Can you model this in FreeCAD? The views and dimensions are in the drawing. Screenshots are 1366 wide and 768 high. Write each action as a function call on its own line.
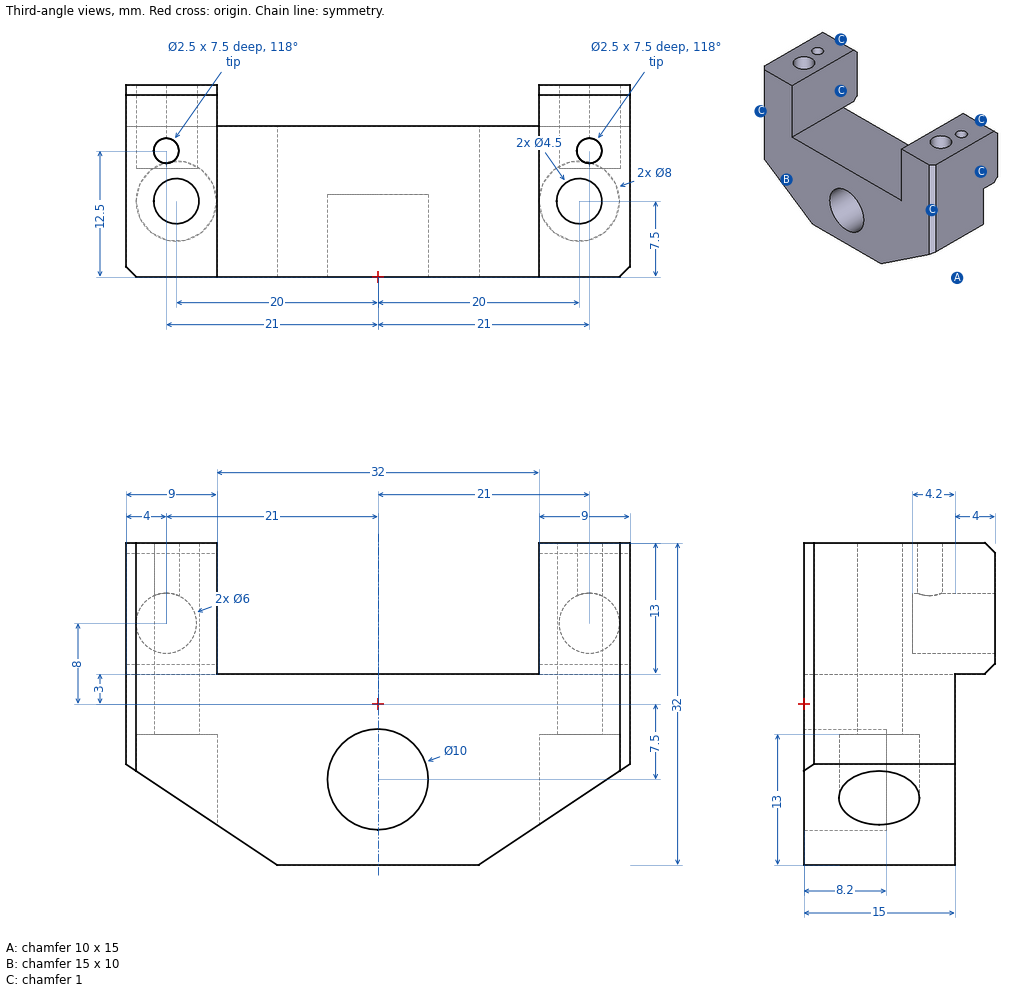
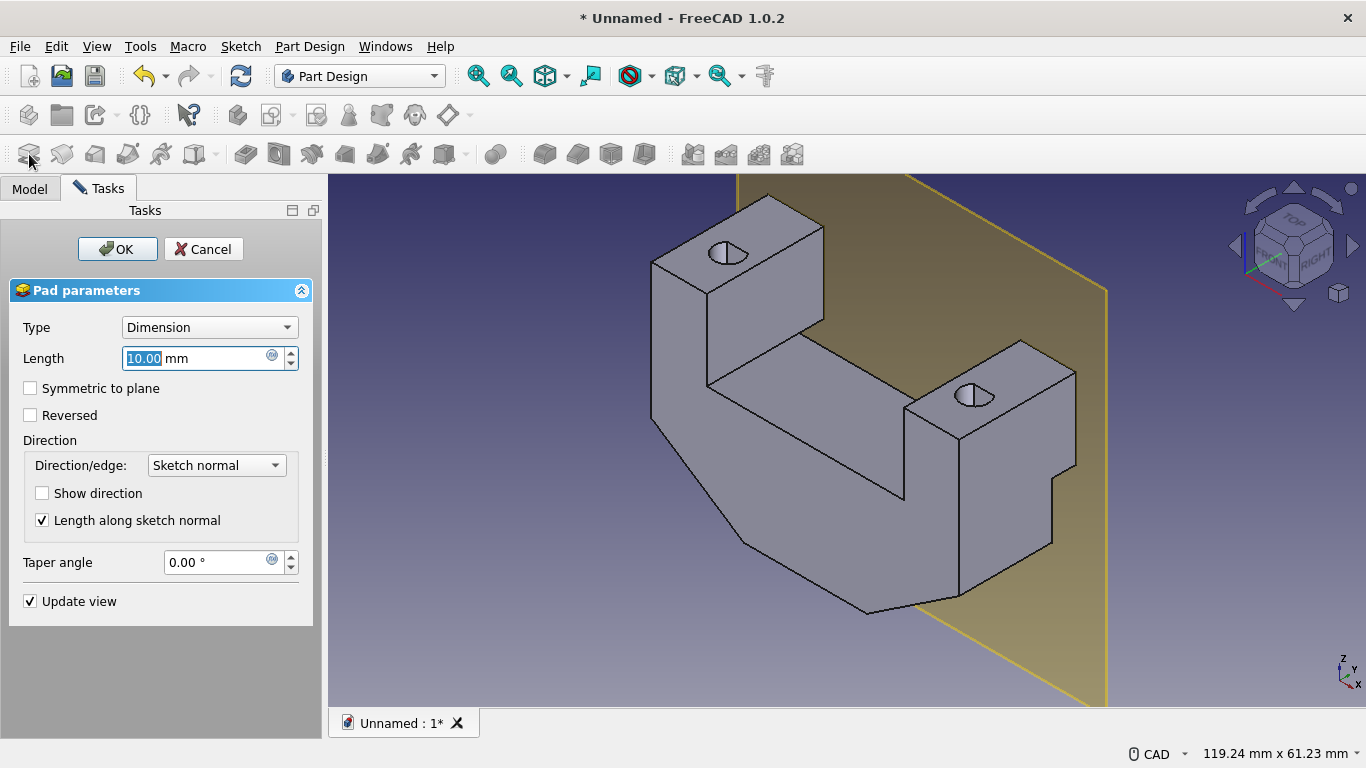
text(4)
key(Tab)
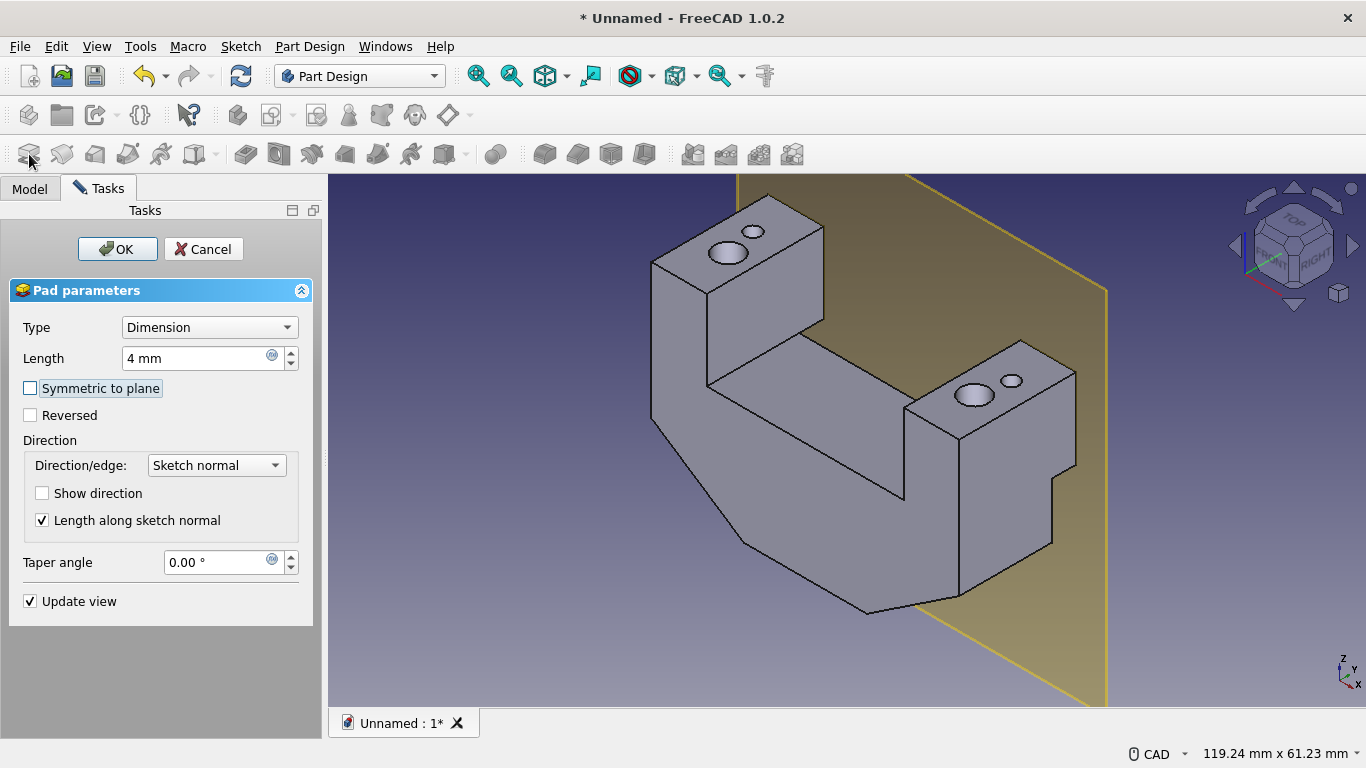
click(118, 249)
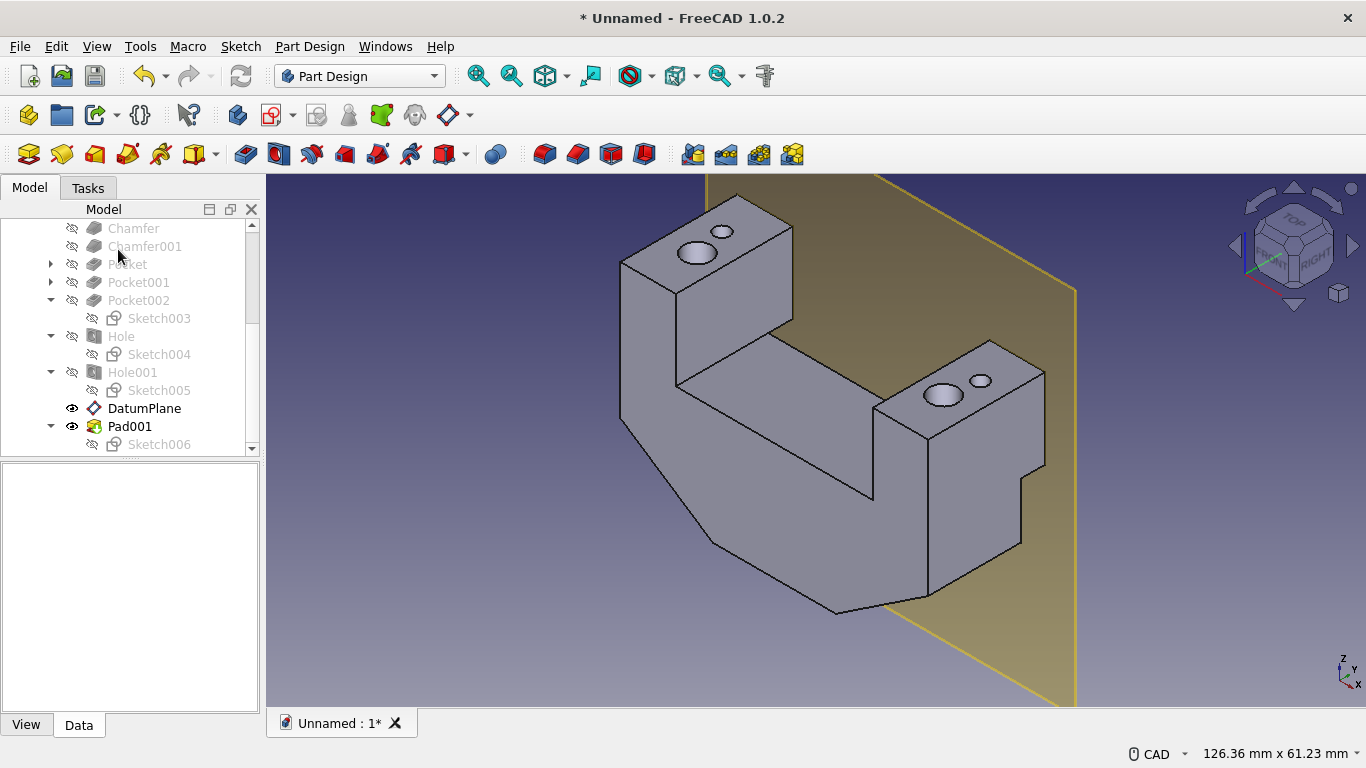
click(117, 408)
key(space)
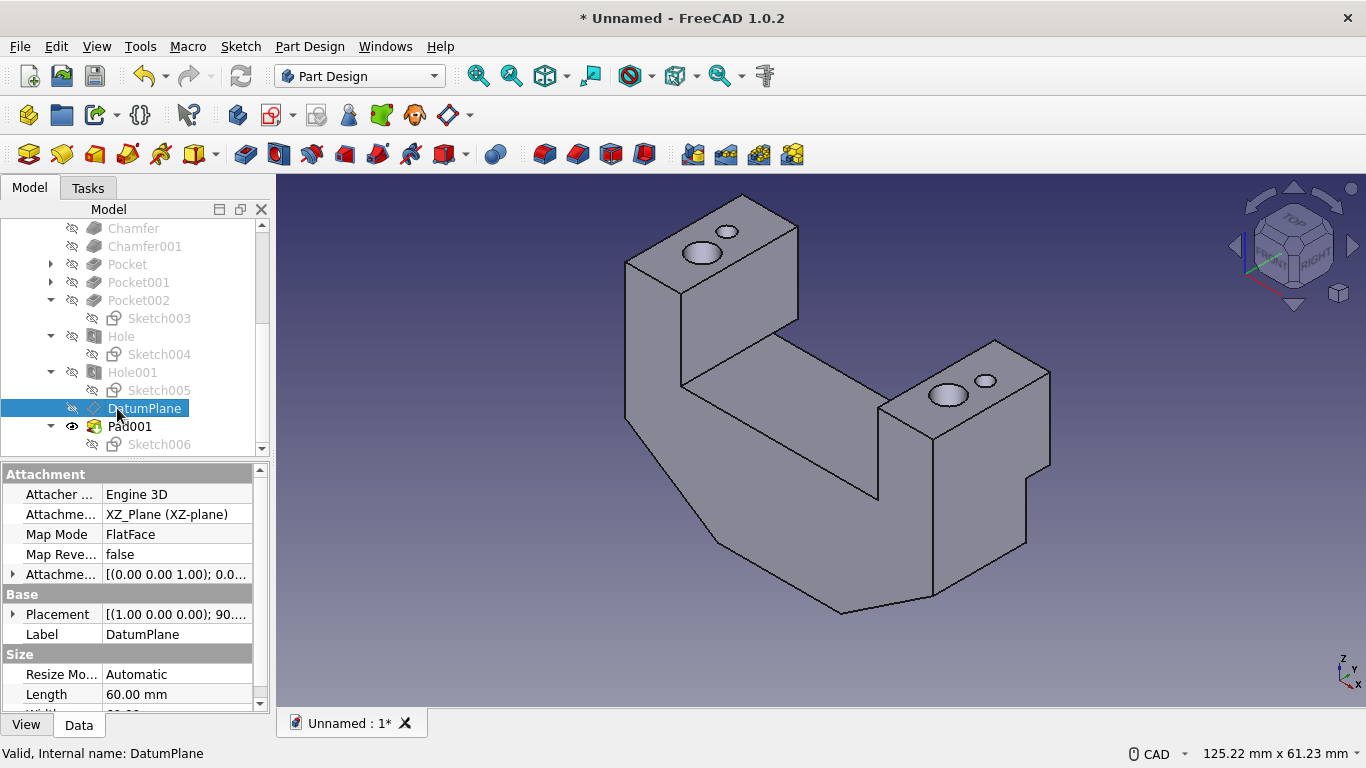
click(823, 521)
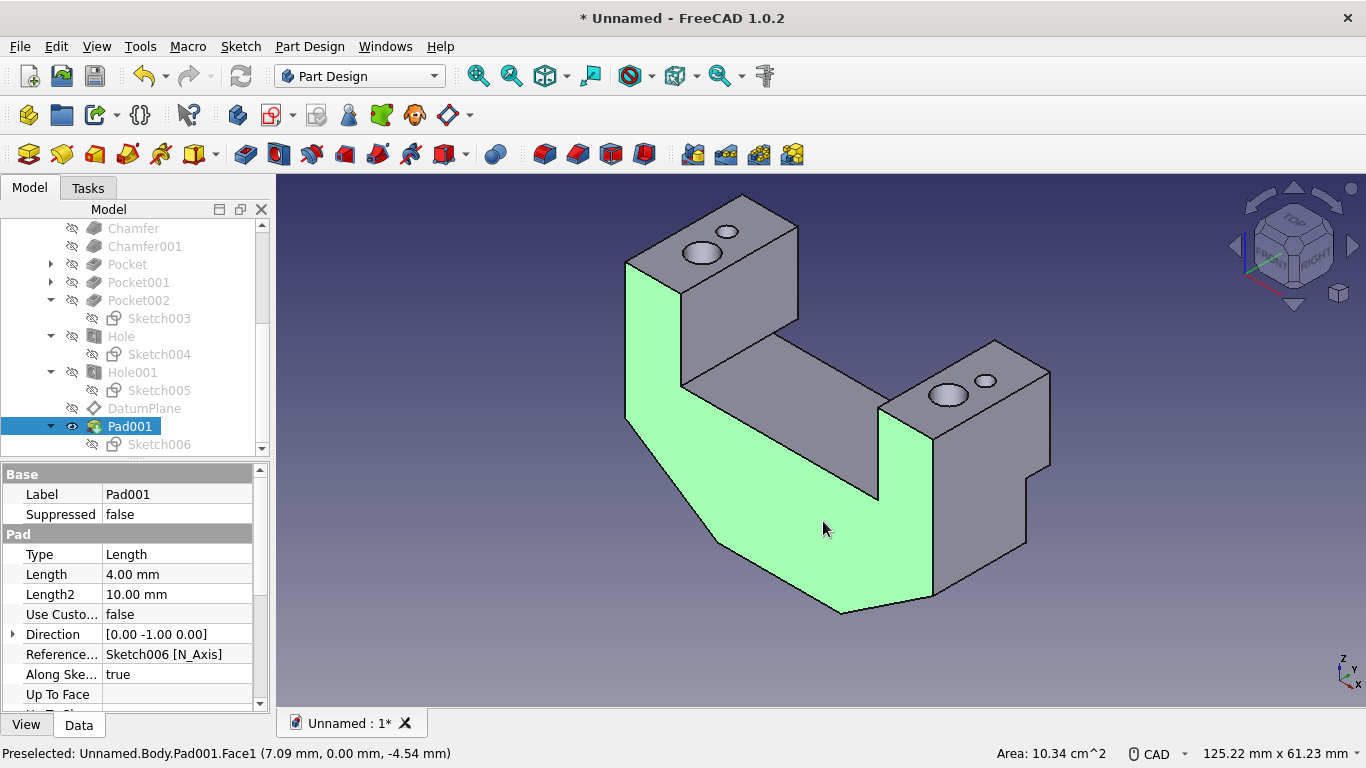
click(270, 116)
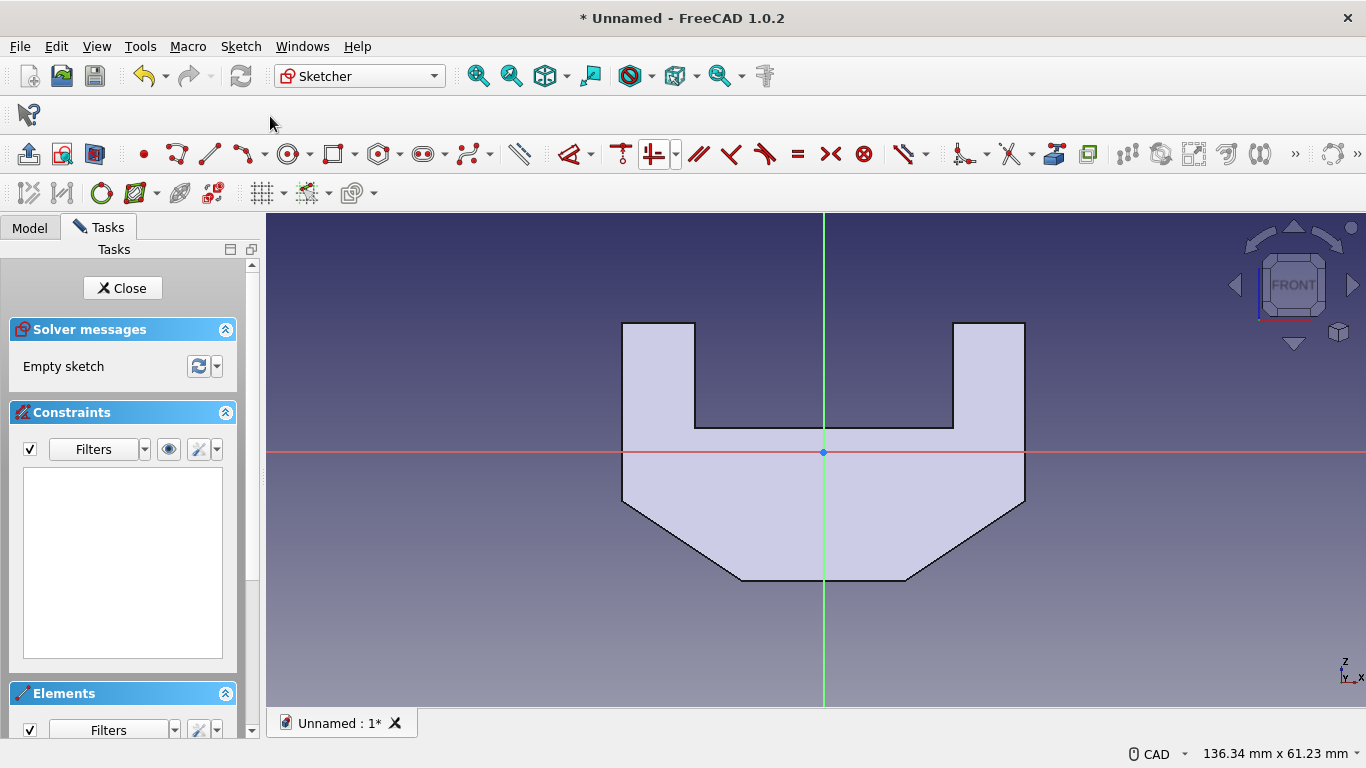
scroll(856, 521, up, 6)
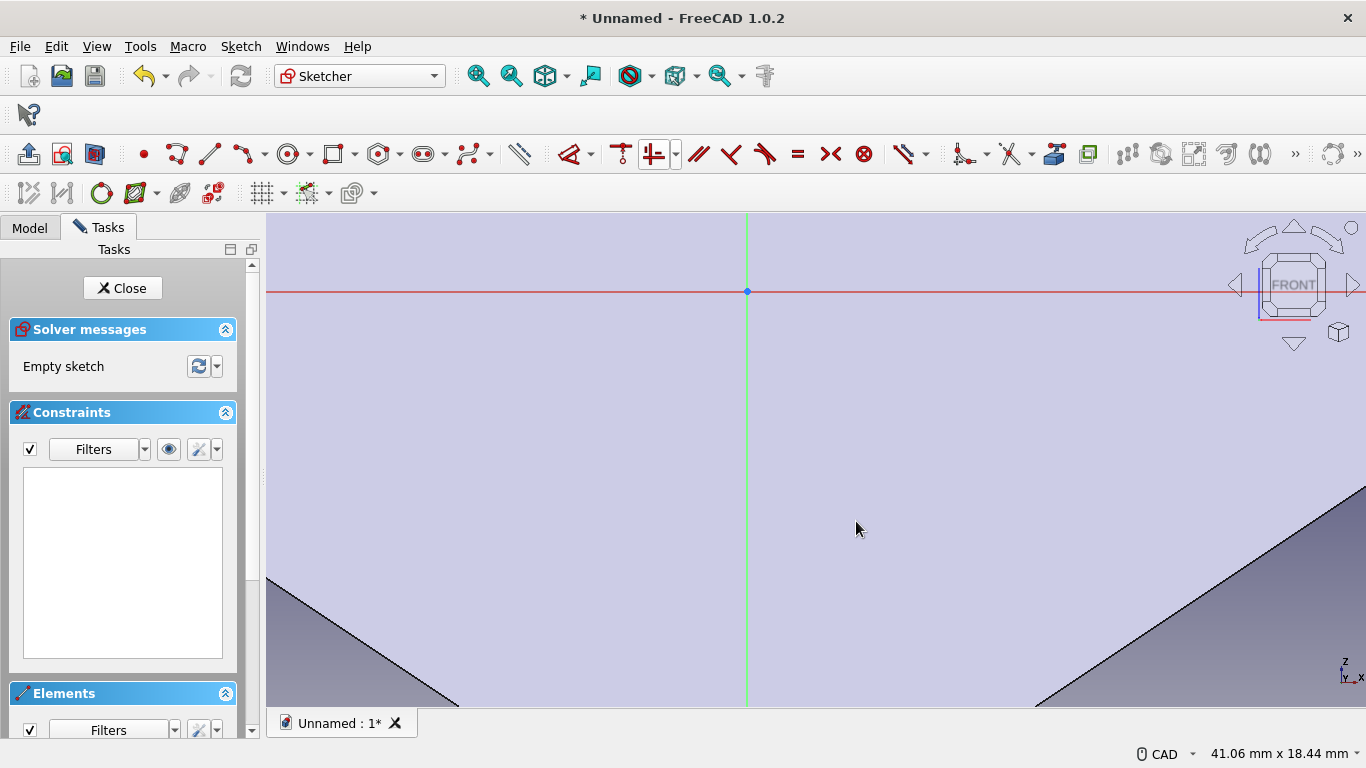
click(288, 154)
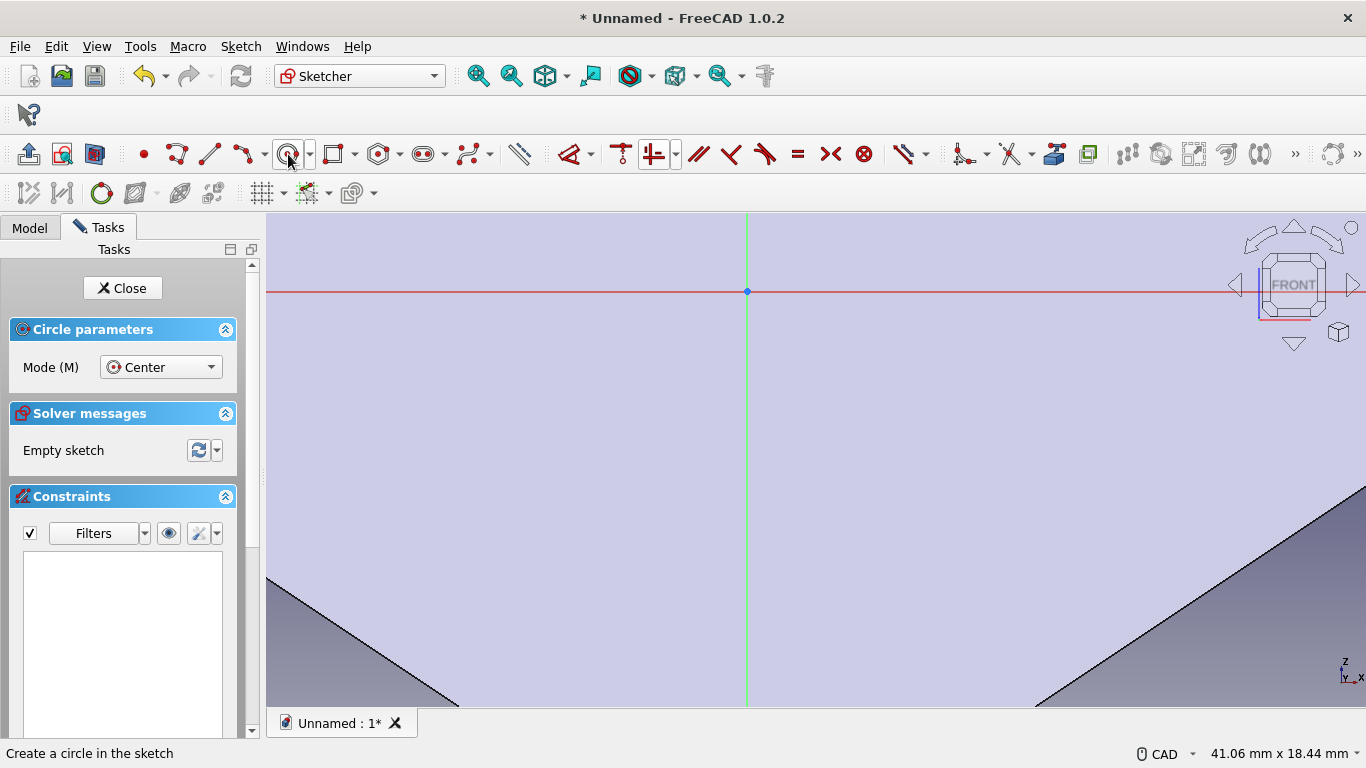
click(747, 493)
move(842, 398)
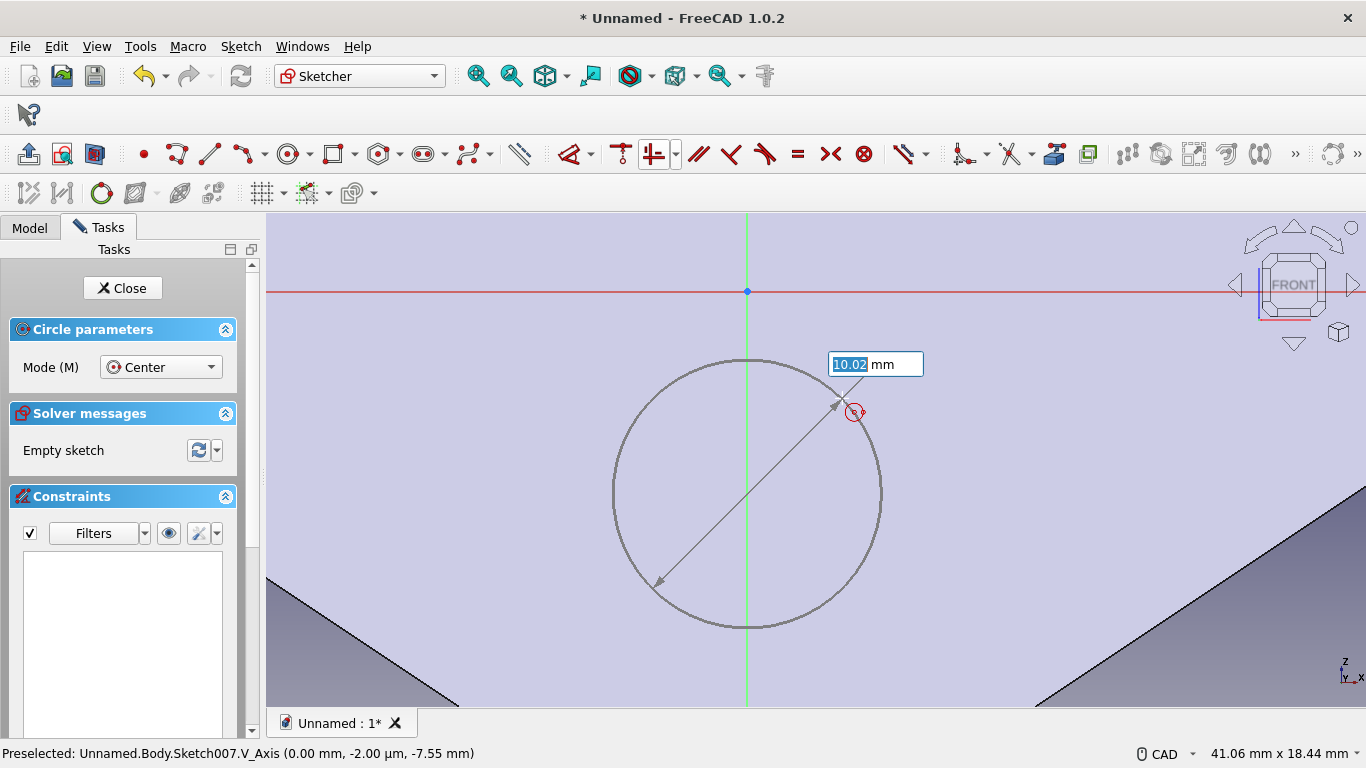
text(10)
key(Return)
key(Escape)